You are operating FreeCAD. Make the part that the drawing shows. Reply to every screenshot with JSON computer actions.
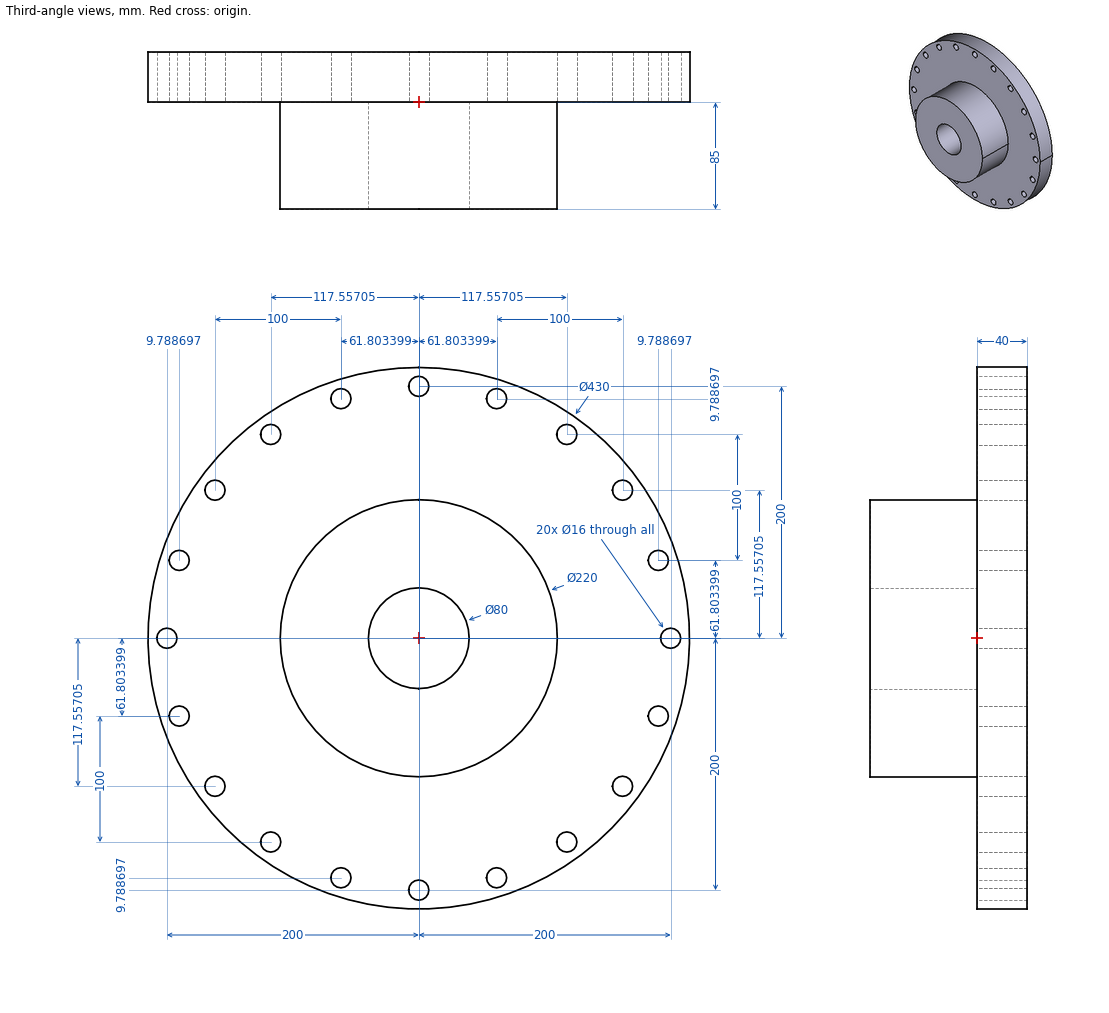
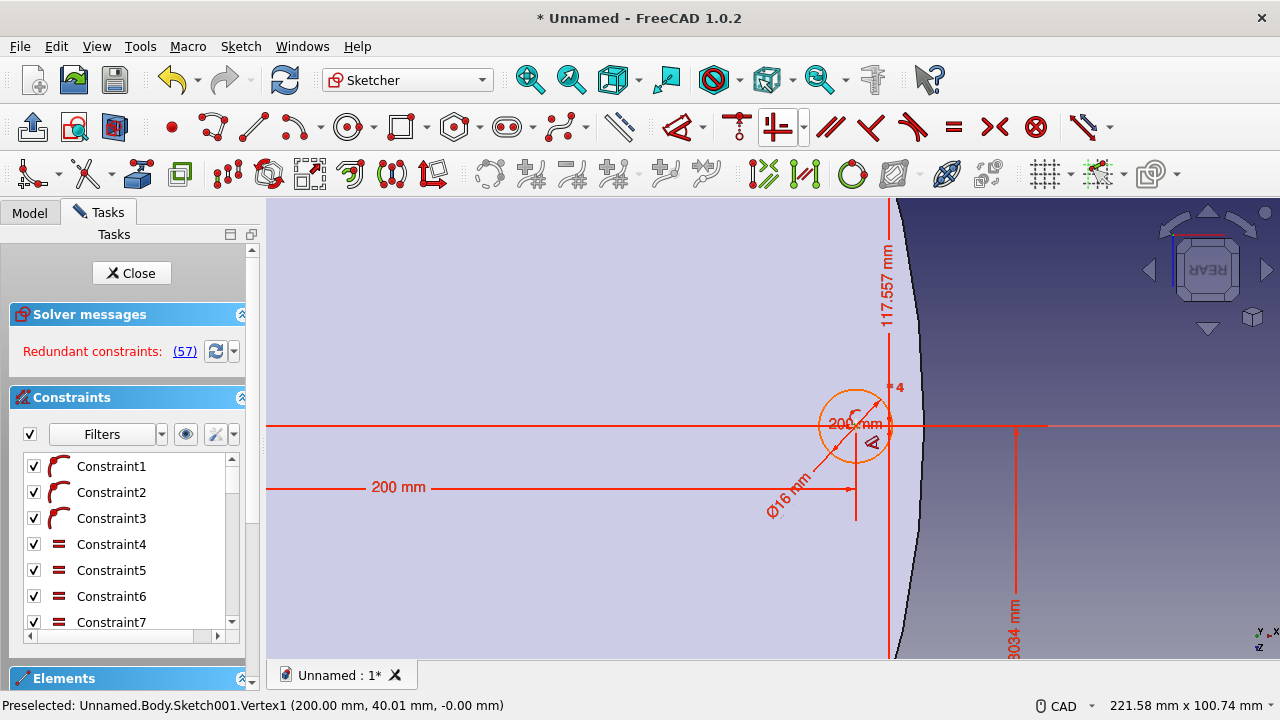
{"action": "scroll", "coordinate": [856, 429], "scroll_direction": "down", "scroll_amount": 9}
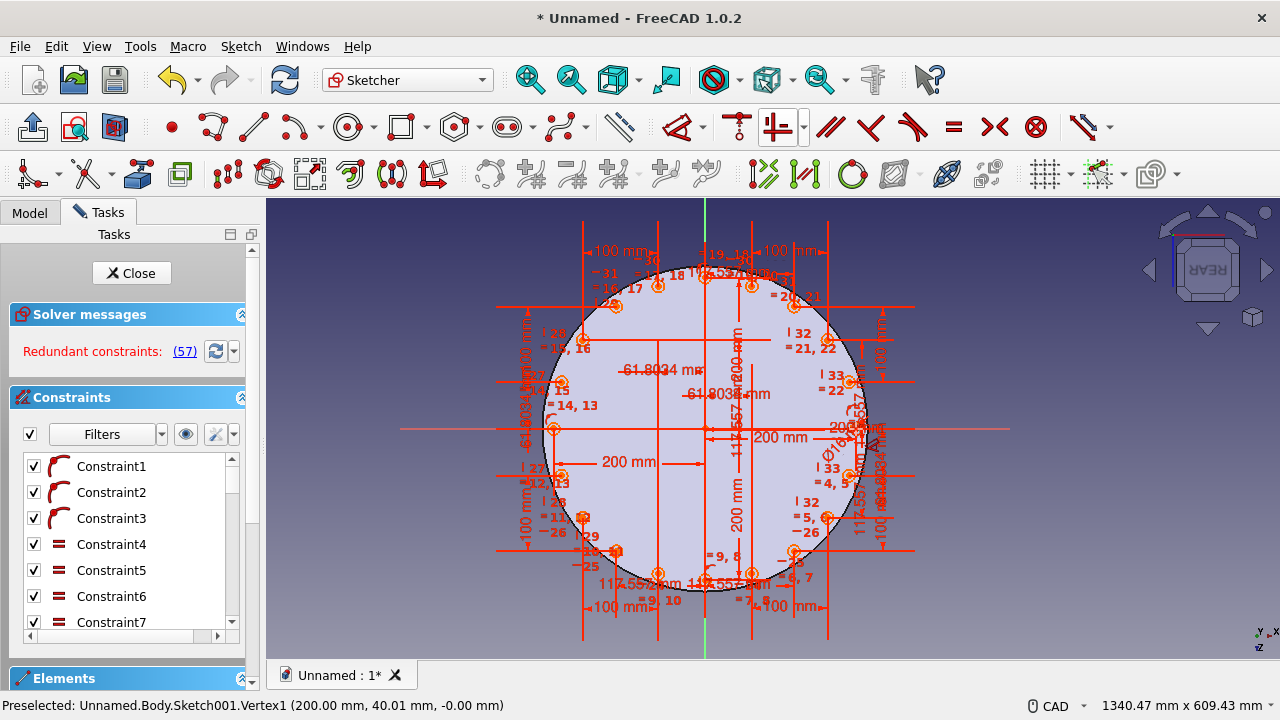
{"action": "scroll", "coordinate": [849, 476], "scroll_direction": "up", "scroll_amount": 9}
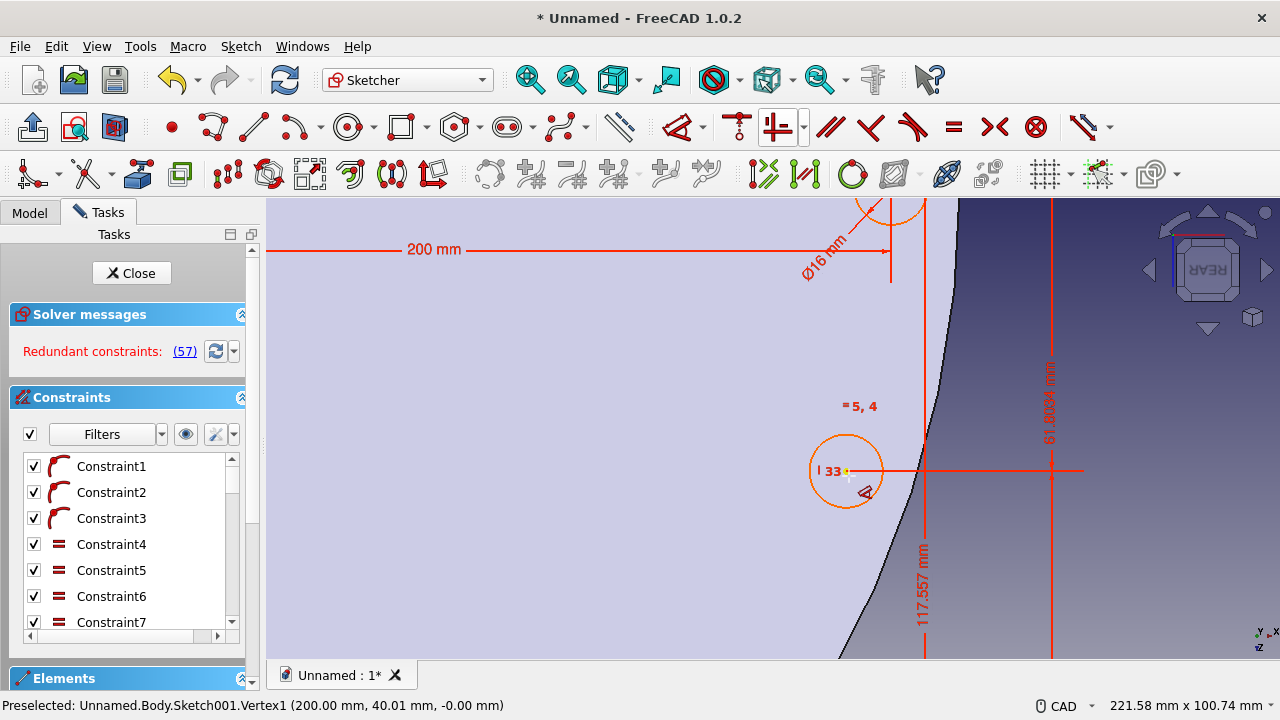
{"action": "left_click", "coordinate": [846, 471]}
{"action": "left_click", "coordinate": [884, 505]}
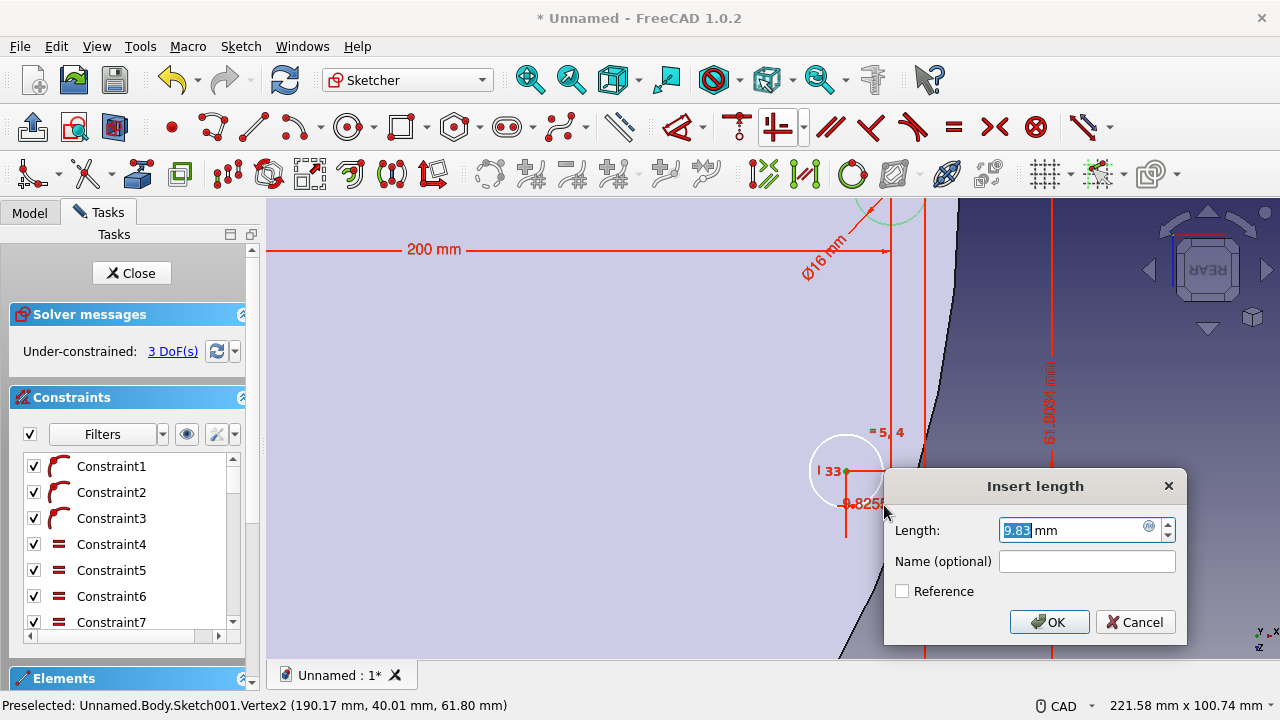
{"action": "type", "text": "9.788697"}
{"action": "key", "text": "Return"}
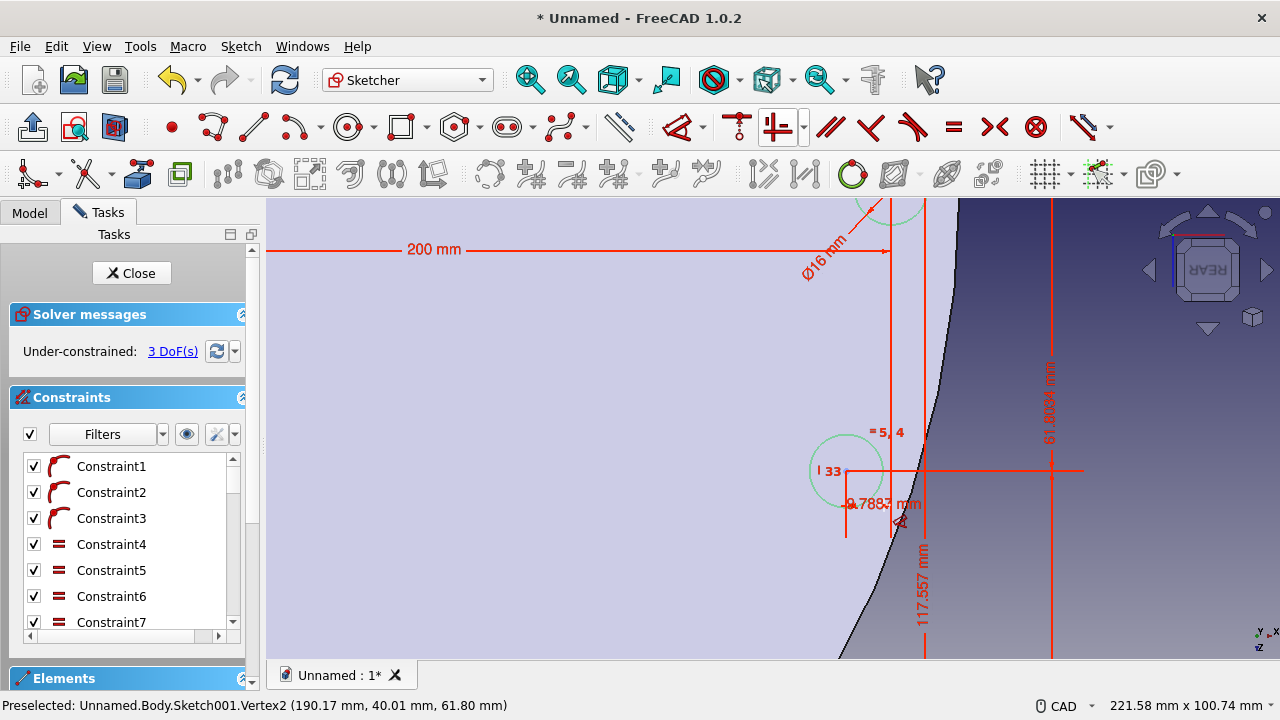
{"action": "scroll", "coordinate": [849, 476], "scroll_direction": "down", "scroll_amount": 9}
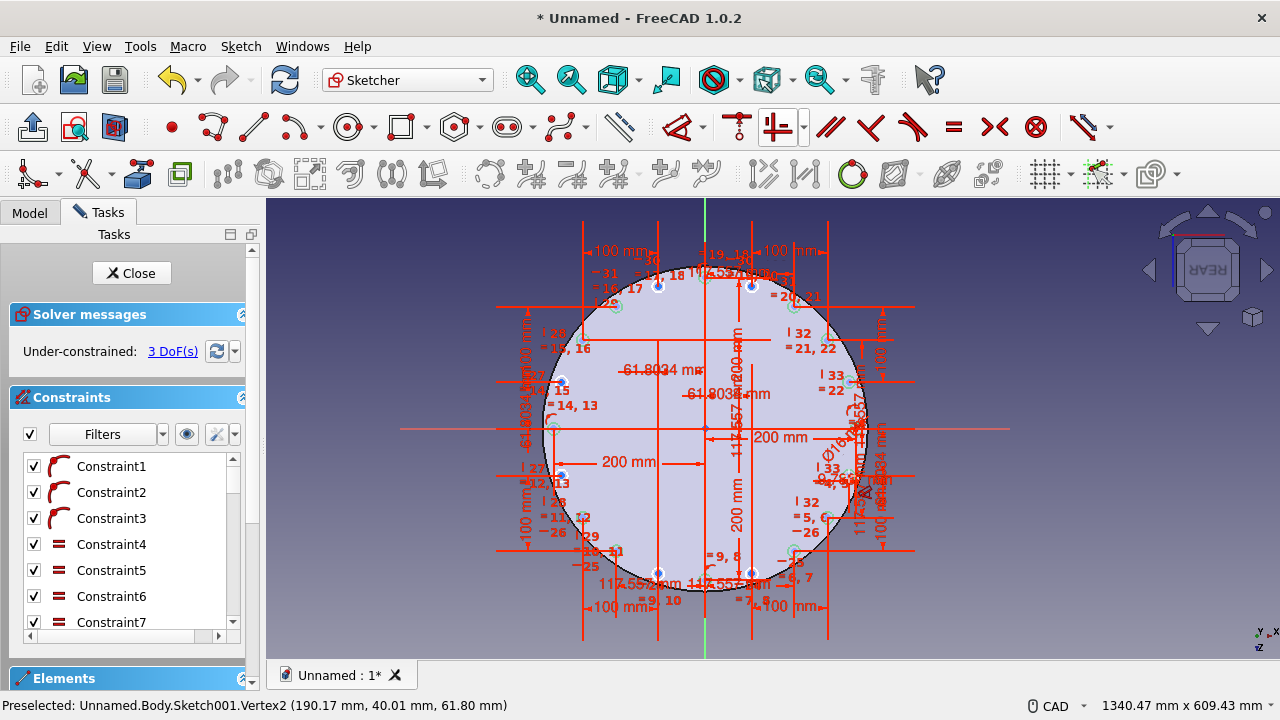
{"action": "scroll", "coordinate": [752, 574], "scroll_direction": "up", "scroll_amount": 9}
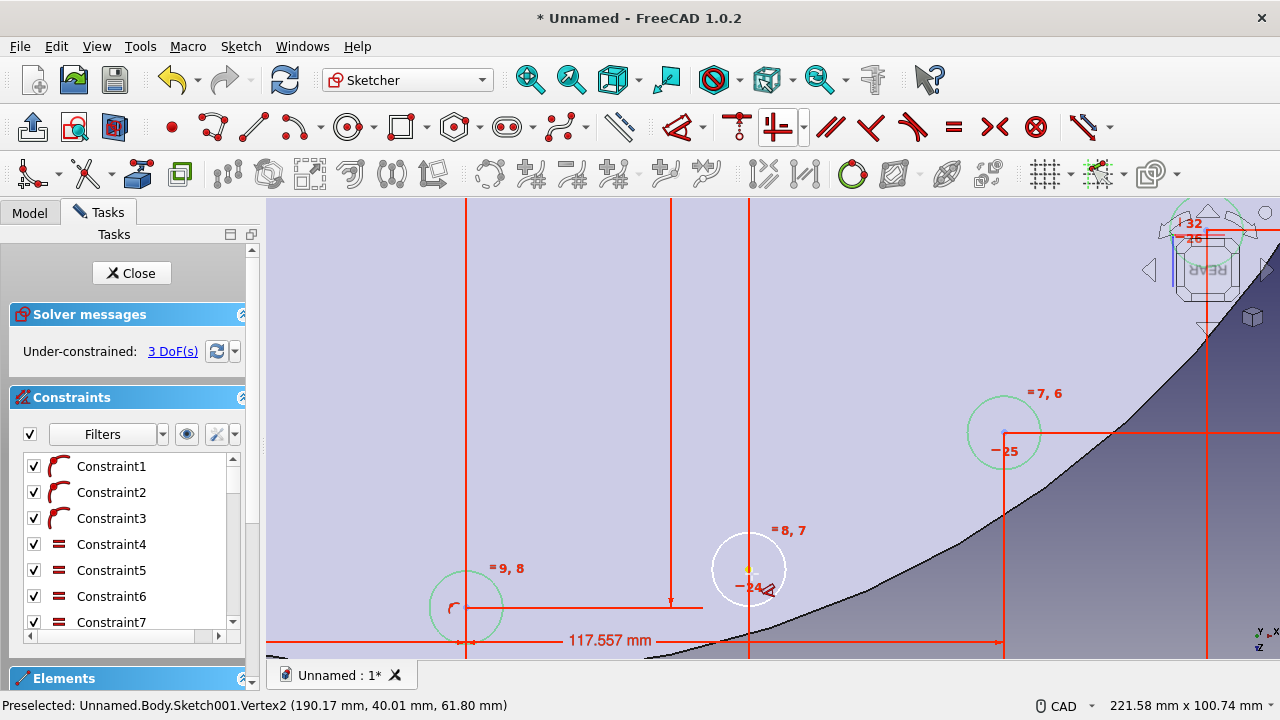
{"action": "left_click", "coordinate": [749, 569]}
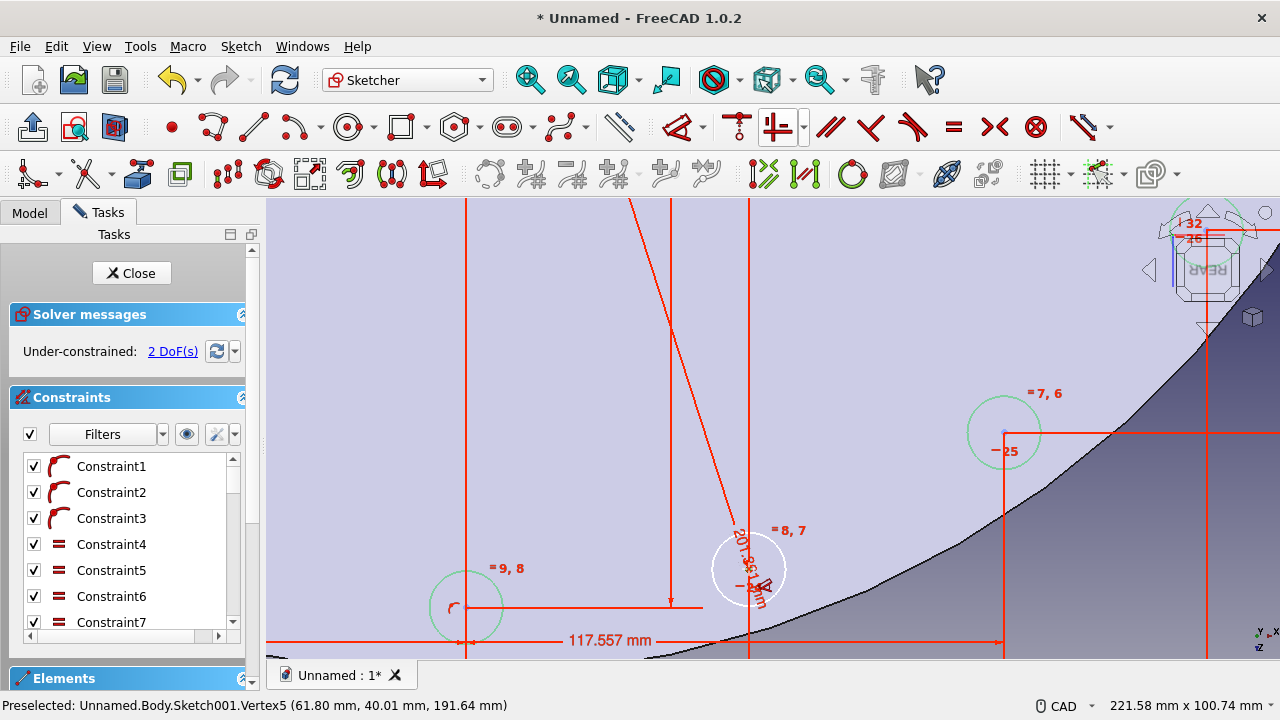
{"action": "left_click", "coordinate": [466, 608]}
{"action": "left_click", "coordinate": [807, 589]}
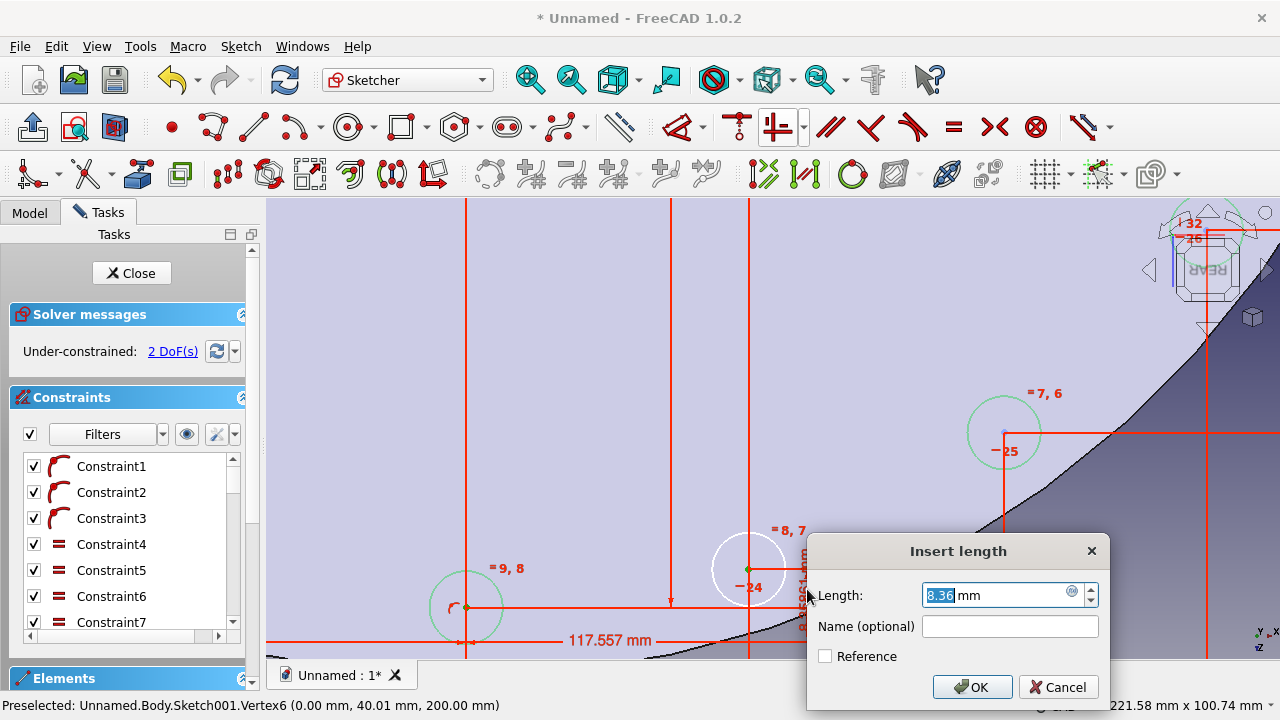
{"action": "type", "text": "9.788697"}
{"action": "key", "text": "Return"}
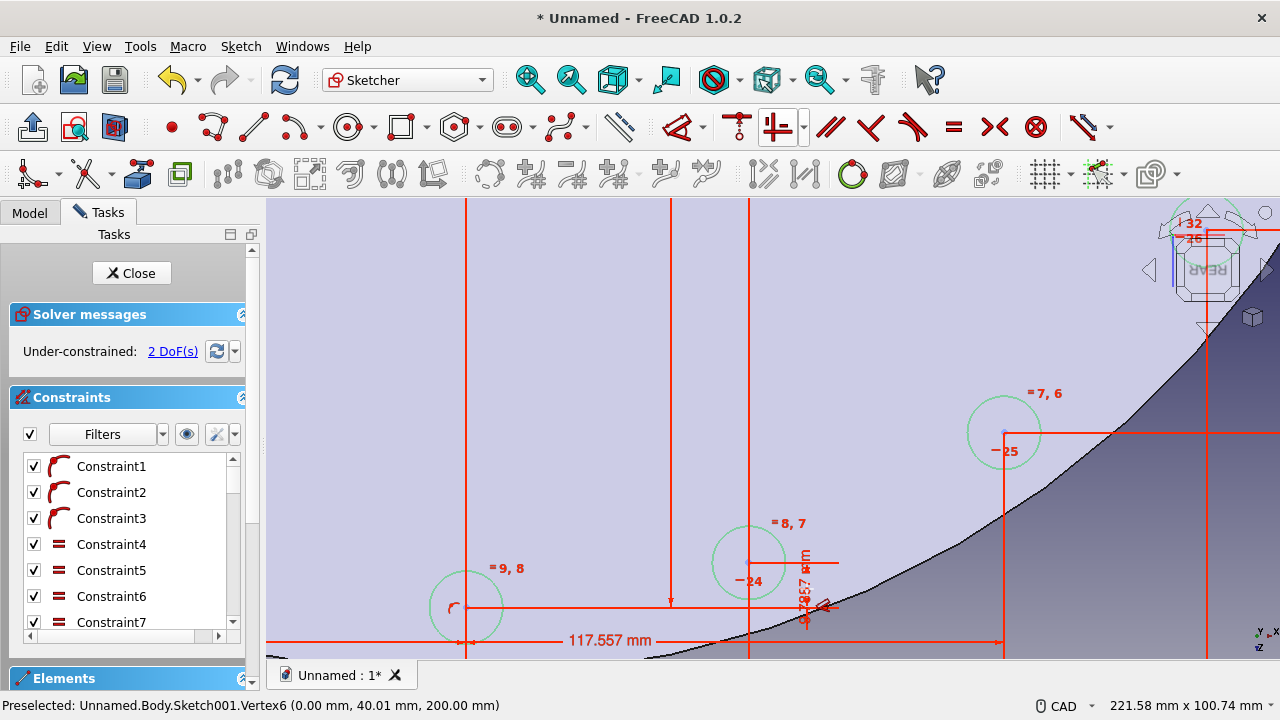
{"action": "scroll", "coordinate": [752, 574], "scroll_direction": "down", "scroll_amount": 9}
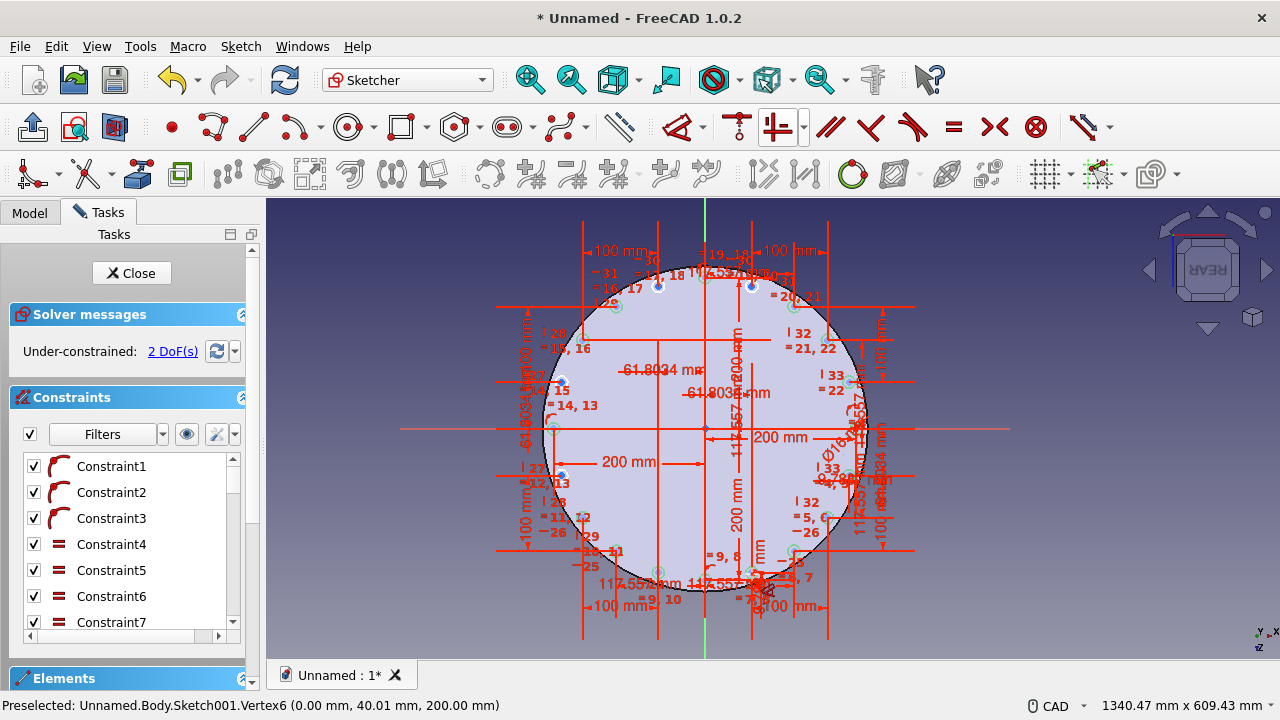
{"action": "scroll", "coordinate": [562, 476], "scroll_direction": "up", "scroll_amount": 9}